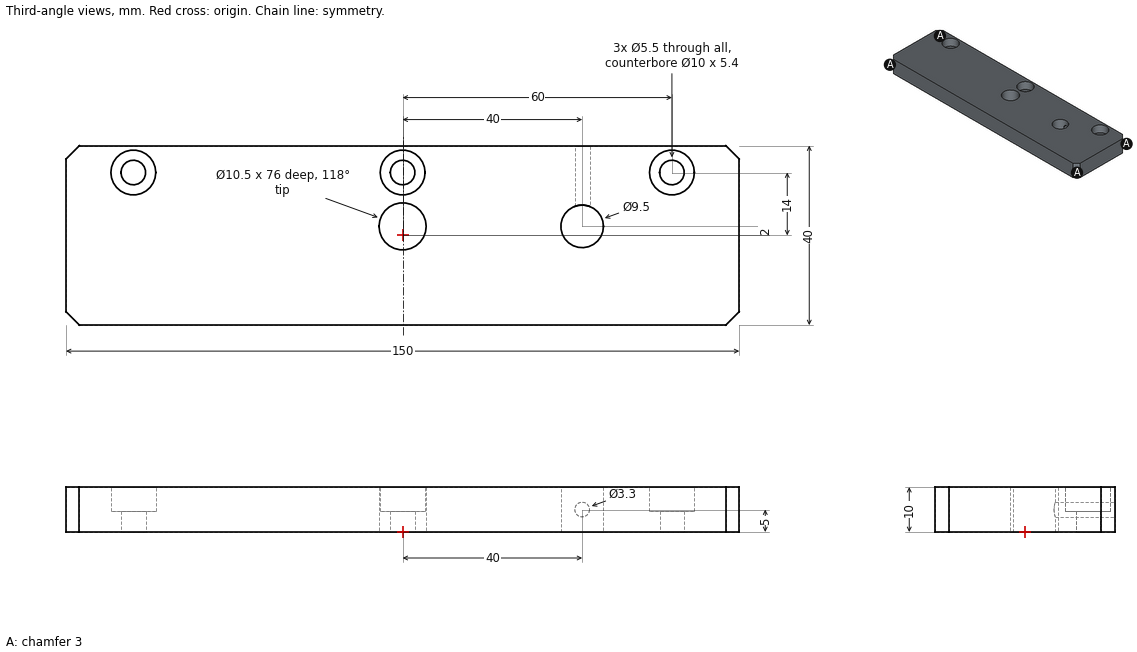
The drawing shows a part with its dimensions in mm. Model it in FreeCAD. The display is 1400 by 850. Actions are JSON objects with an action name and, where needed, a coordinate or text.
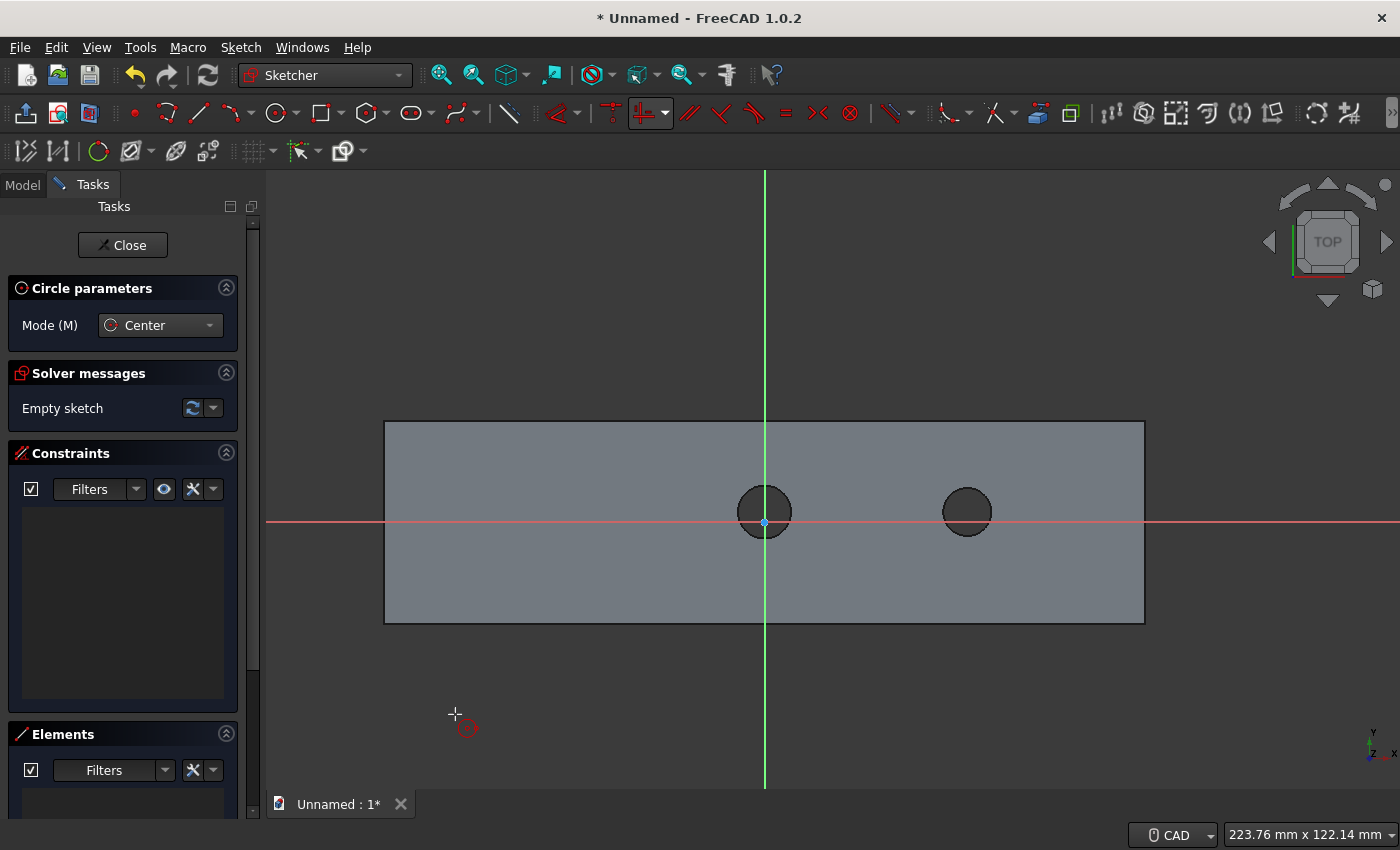
{"action": "scroll", "coordinate": [1069, 451], "scroll_direction": "up", "scroll_amount": 3}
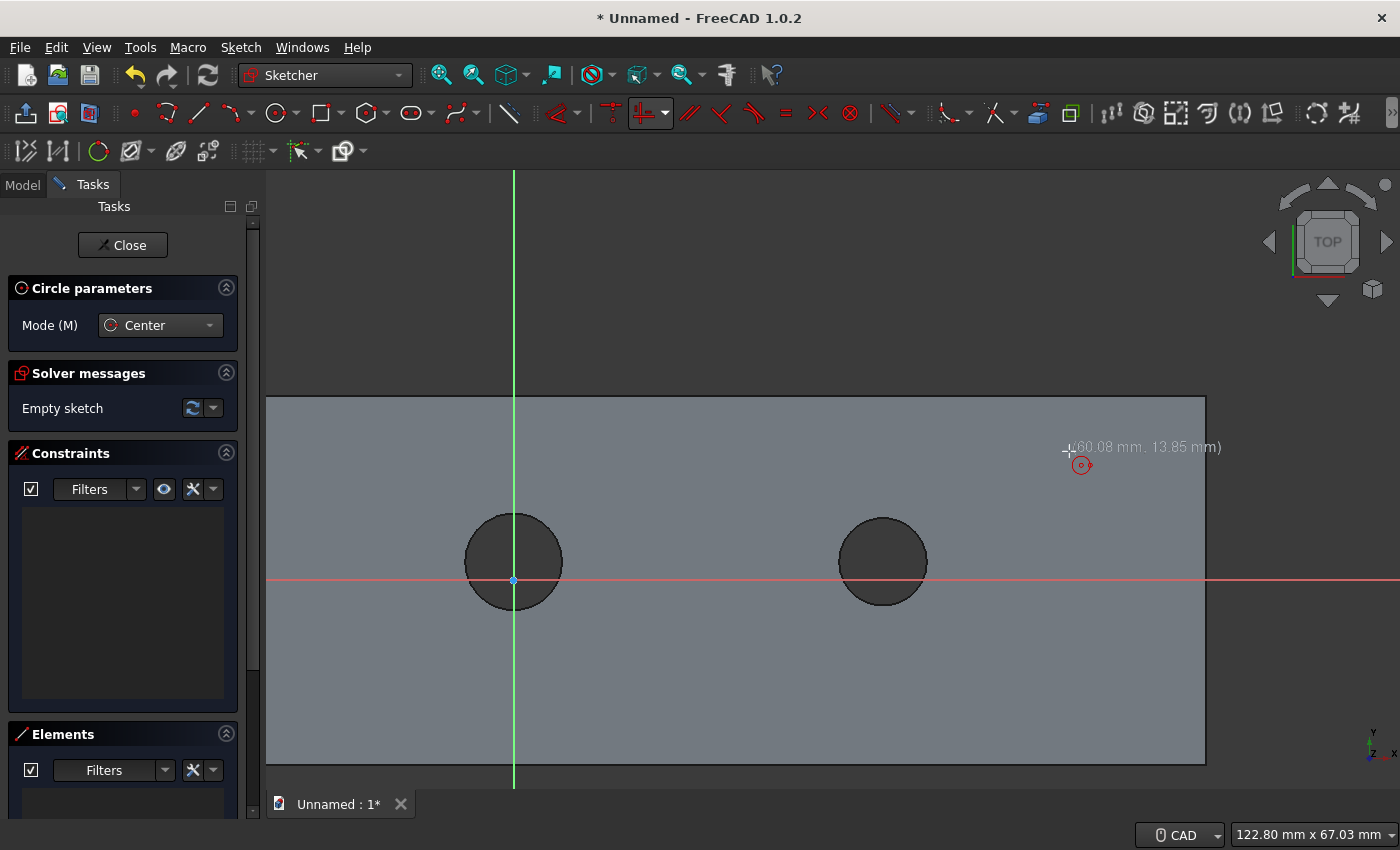
{"action": "left_click", "coordinate": [1068, 451]}
{"action": "mouse_move", "coordinate": [1086, 433]}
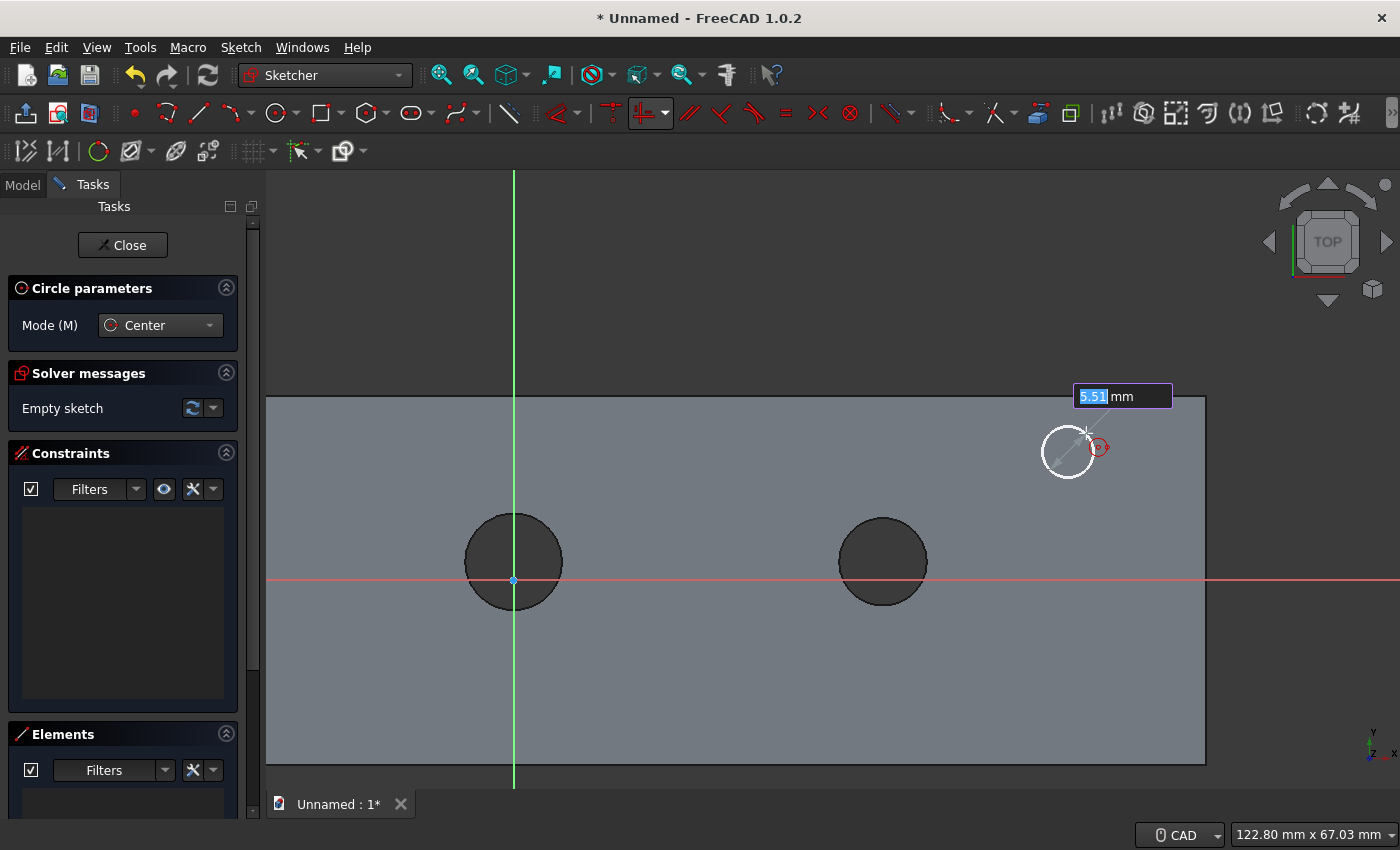
{"action": "type", "text": "5.5"}
{"action": "key", "text": "Return"}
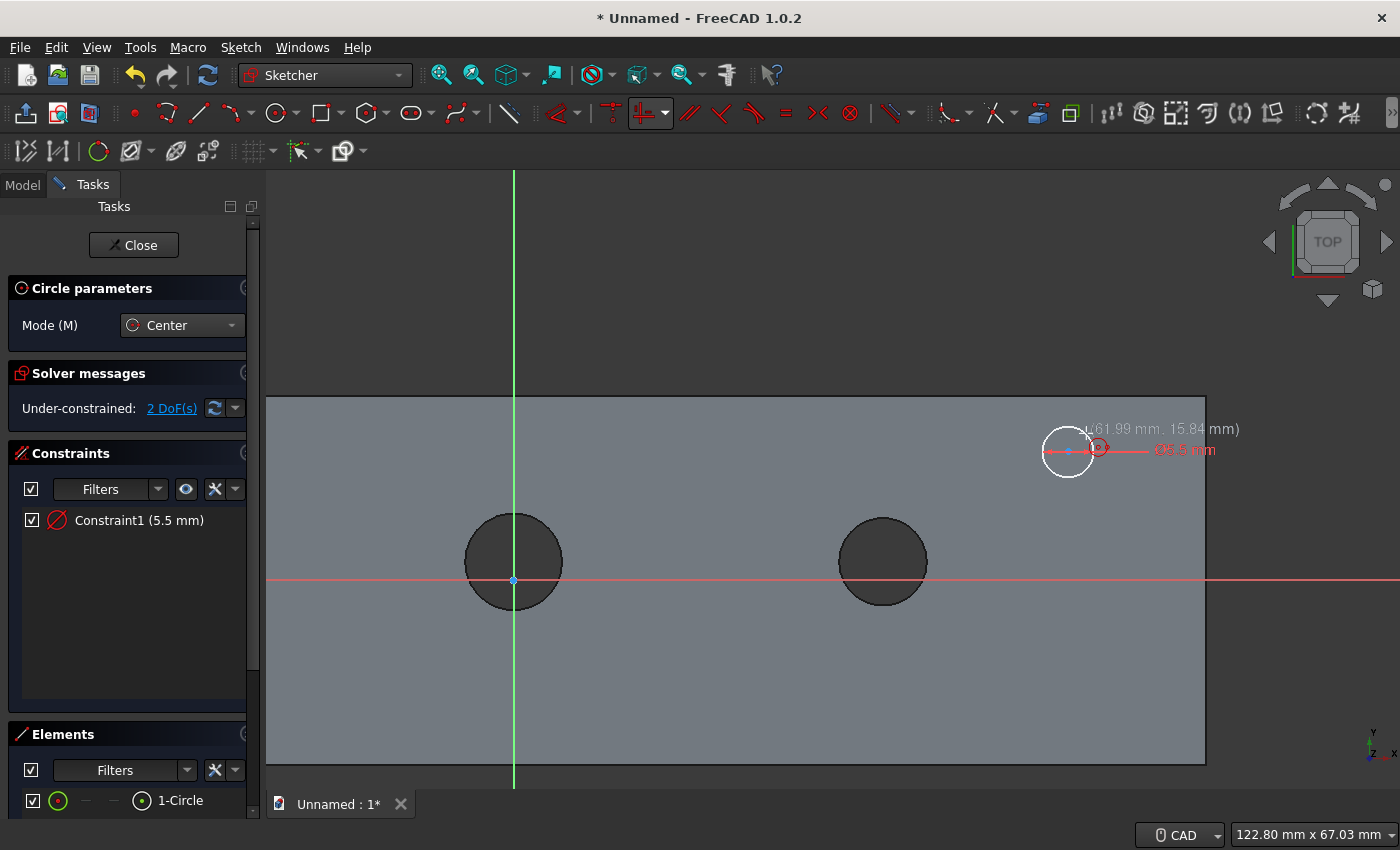
{"action": "left_click", "coordinate": [514, 451]}
{"action": "mouse_move", "coordinate": [532, 433]}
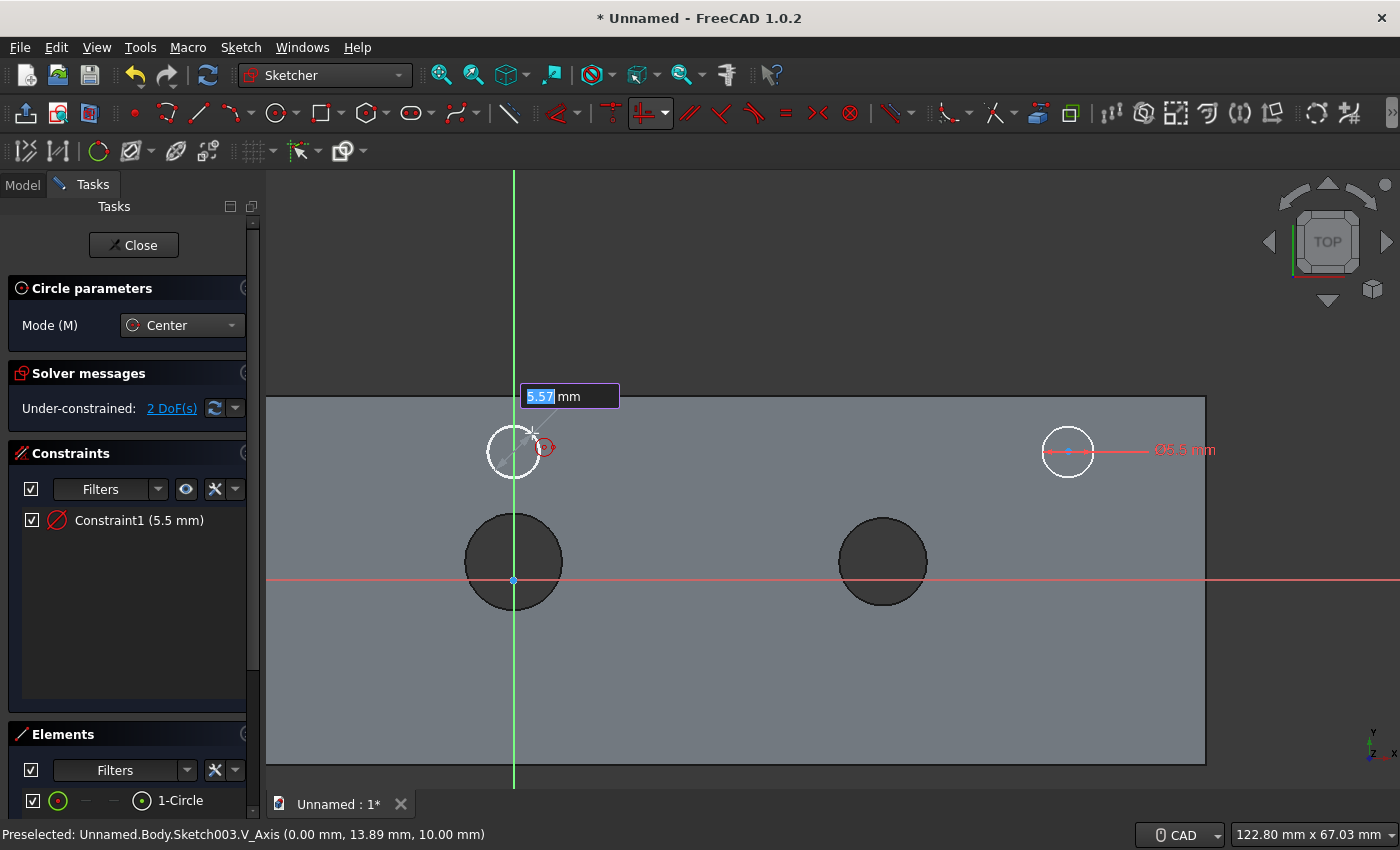
{"action": "type", "text": "5.5"}
{"action": "key", "text": "Return"}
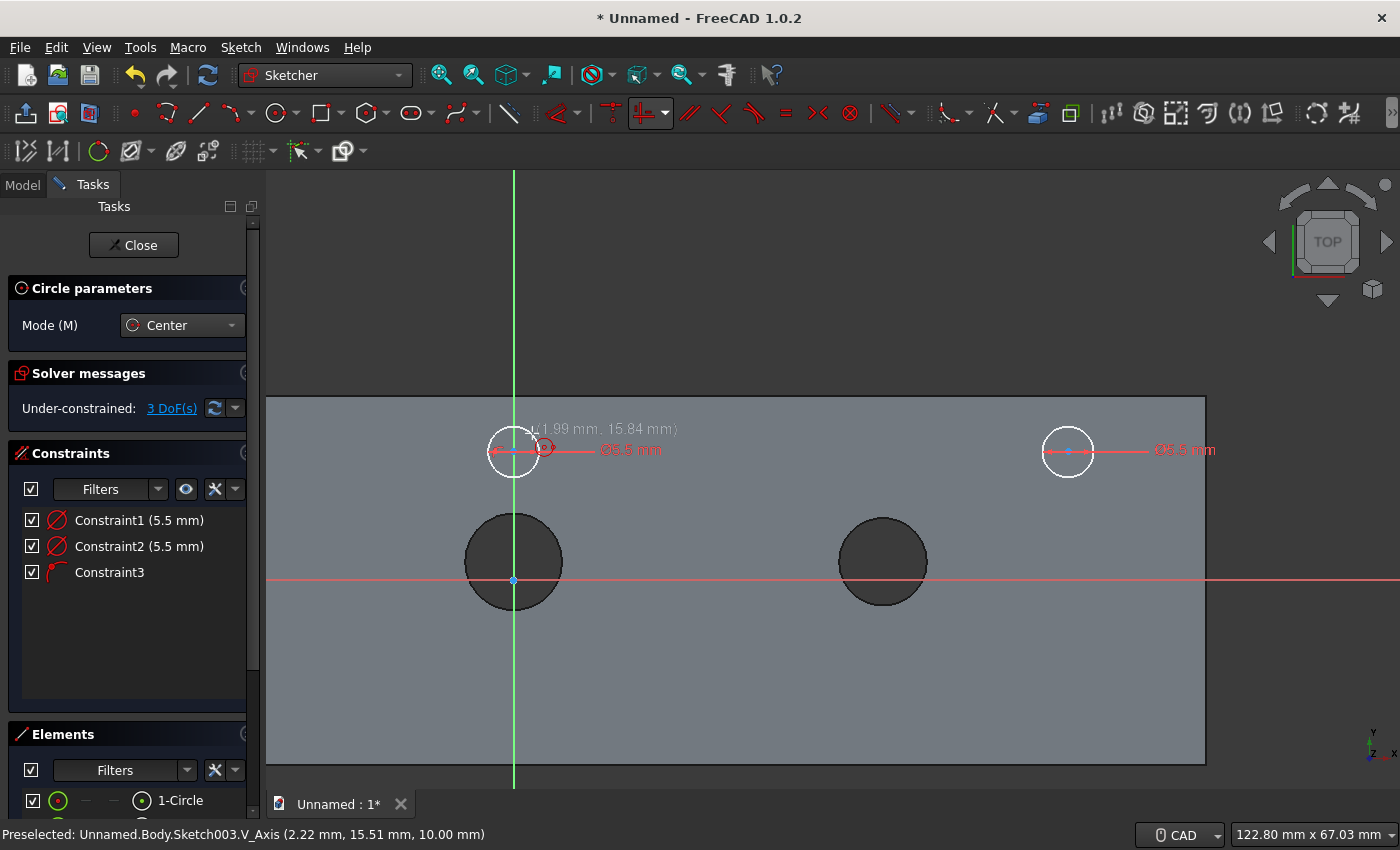
{"action": "scroll", "coordinate": [1070, 451], "scroll_direction": "down", "scroll_amount": 3}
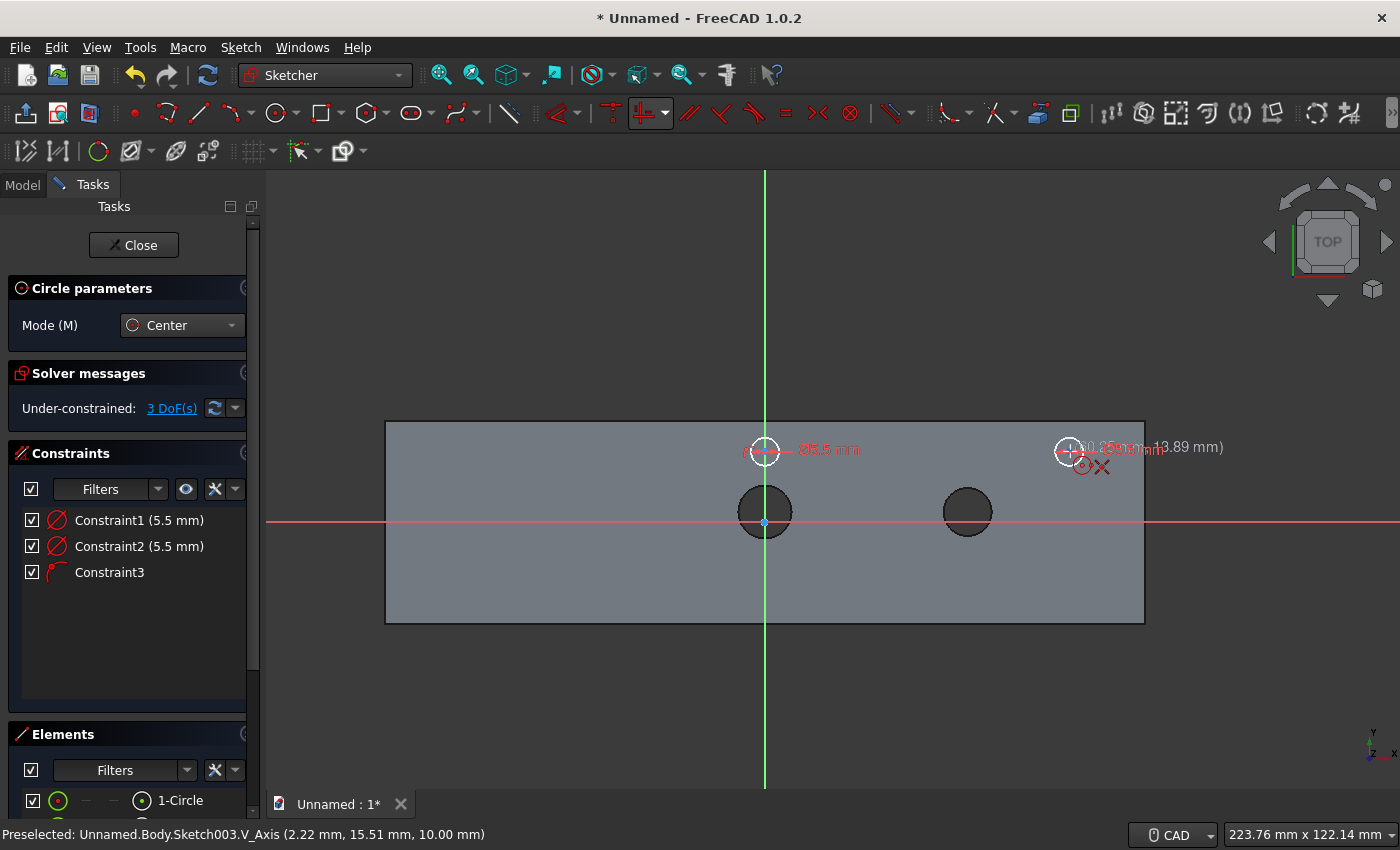
{"action": "scroll", "coordinate": [461, 451], "scroll_direction": "up", "scroll_amount": 3}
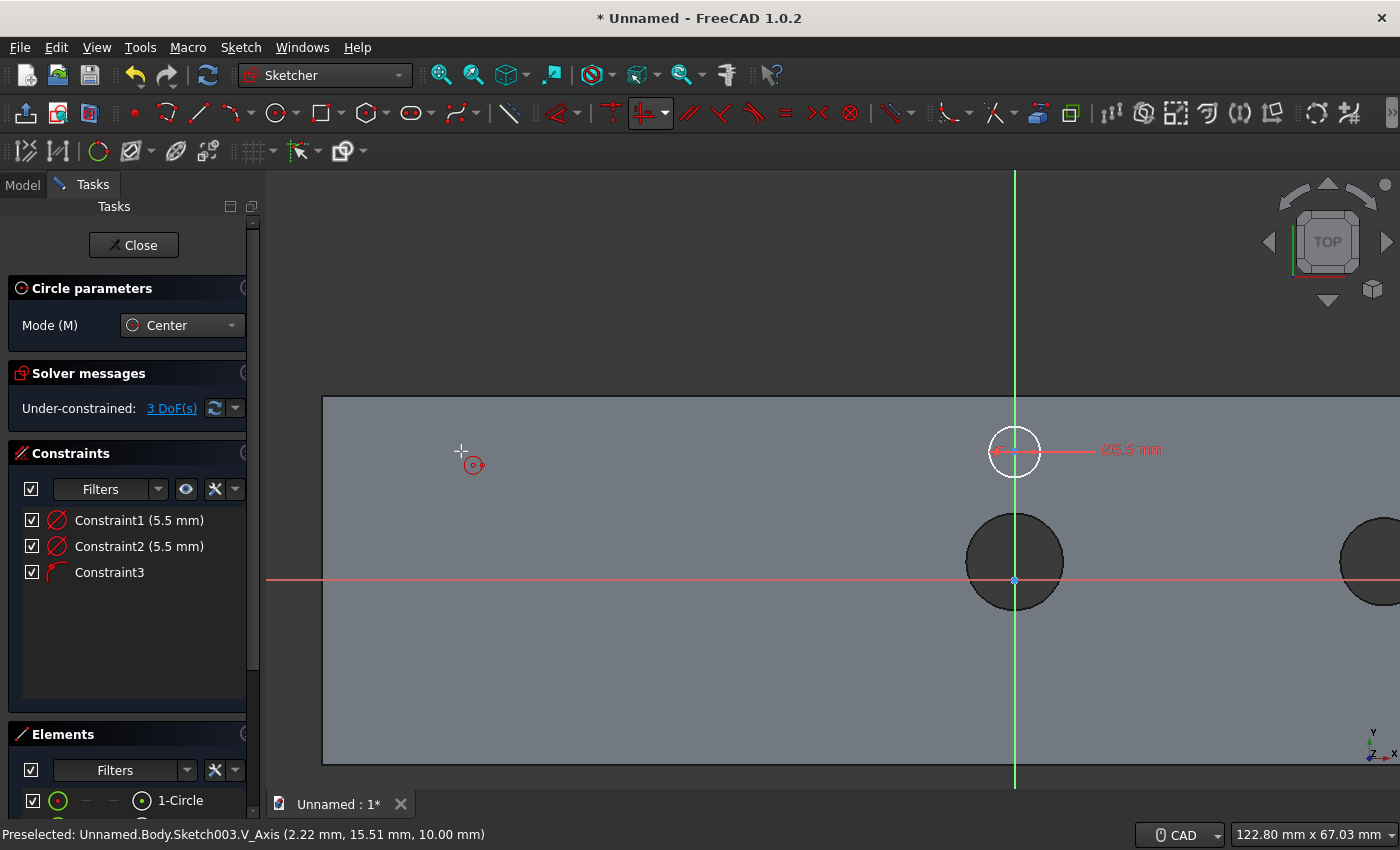
{"action": "left_click", "coordinate": [461, 451]}
{"action": "mouse_move", "coordinate": [479, 433]}